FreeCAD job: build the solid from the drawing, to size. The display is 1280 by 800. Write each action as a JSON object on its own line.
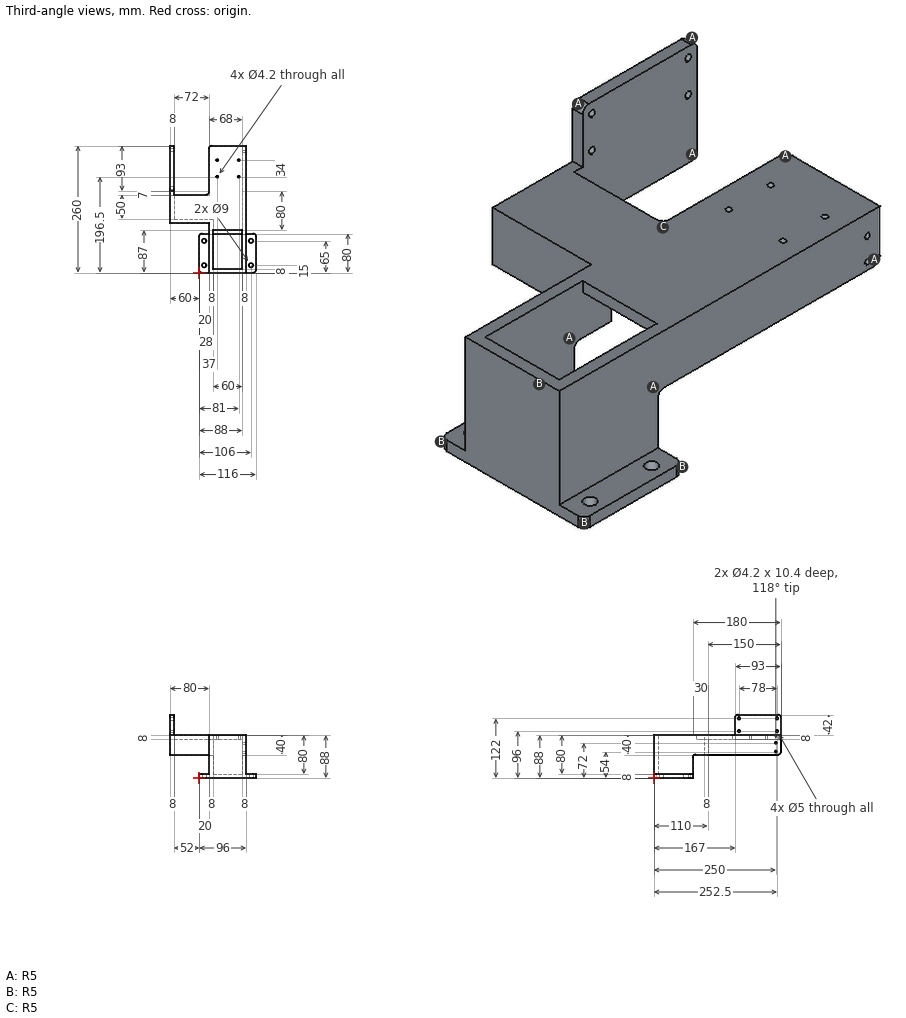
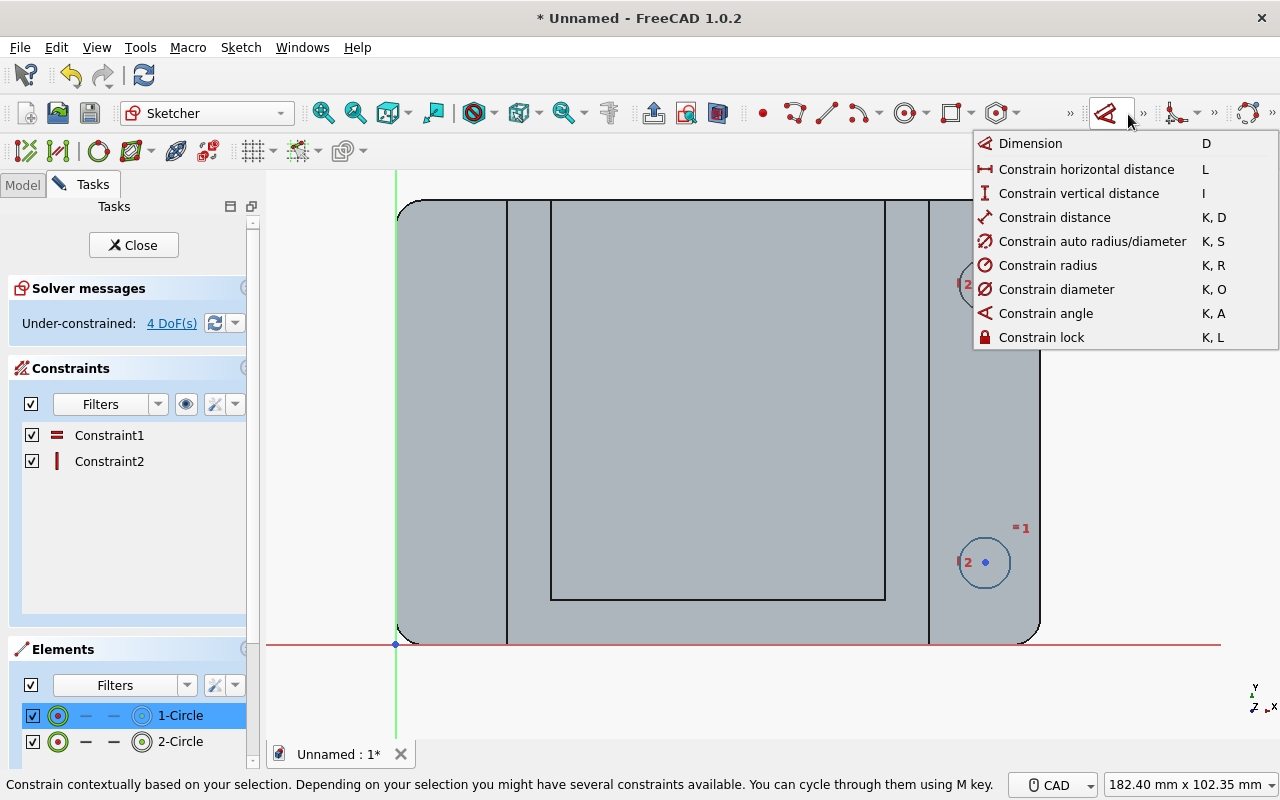
{"action": "left_click", "coordinate": [1126, 289]}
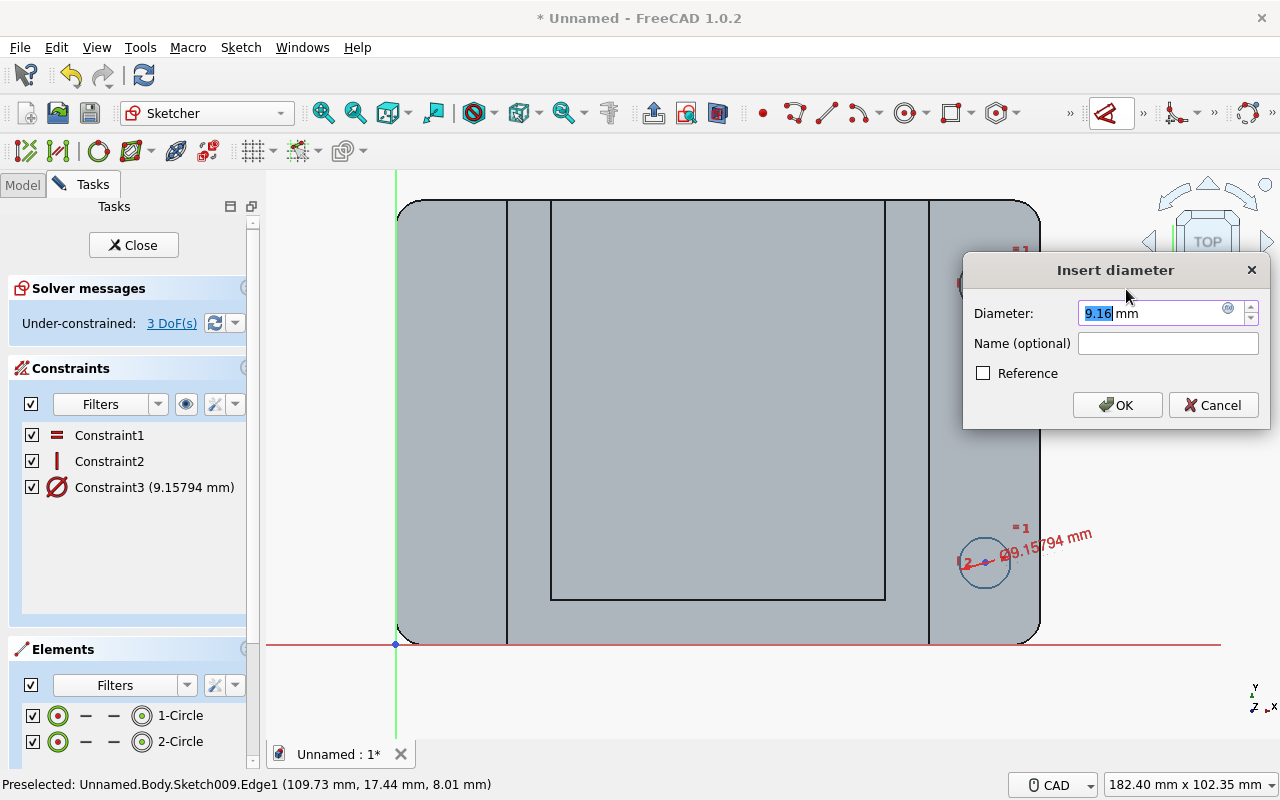
{"action": "type", "text": "9"}
{"action": "key", "text": "Return"}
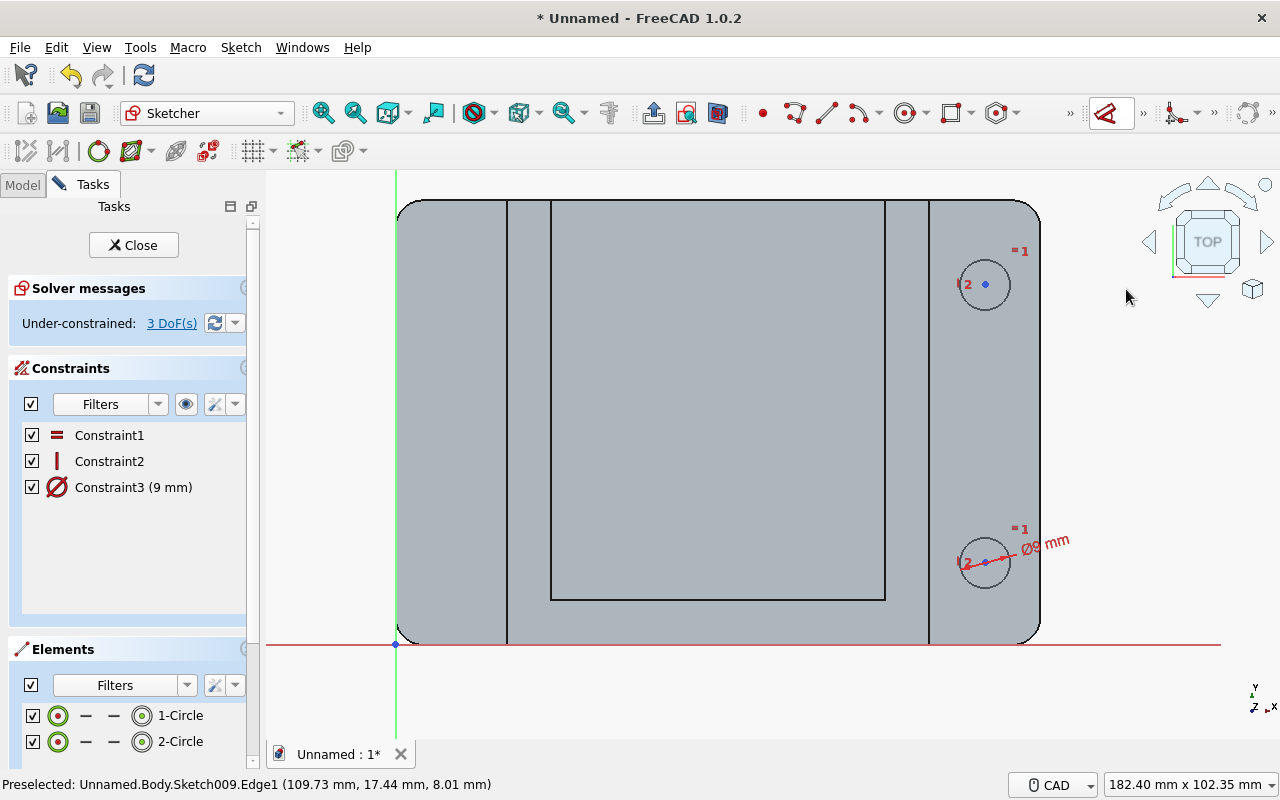
{"action": "left_click", "coordinate": [985, 563]}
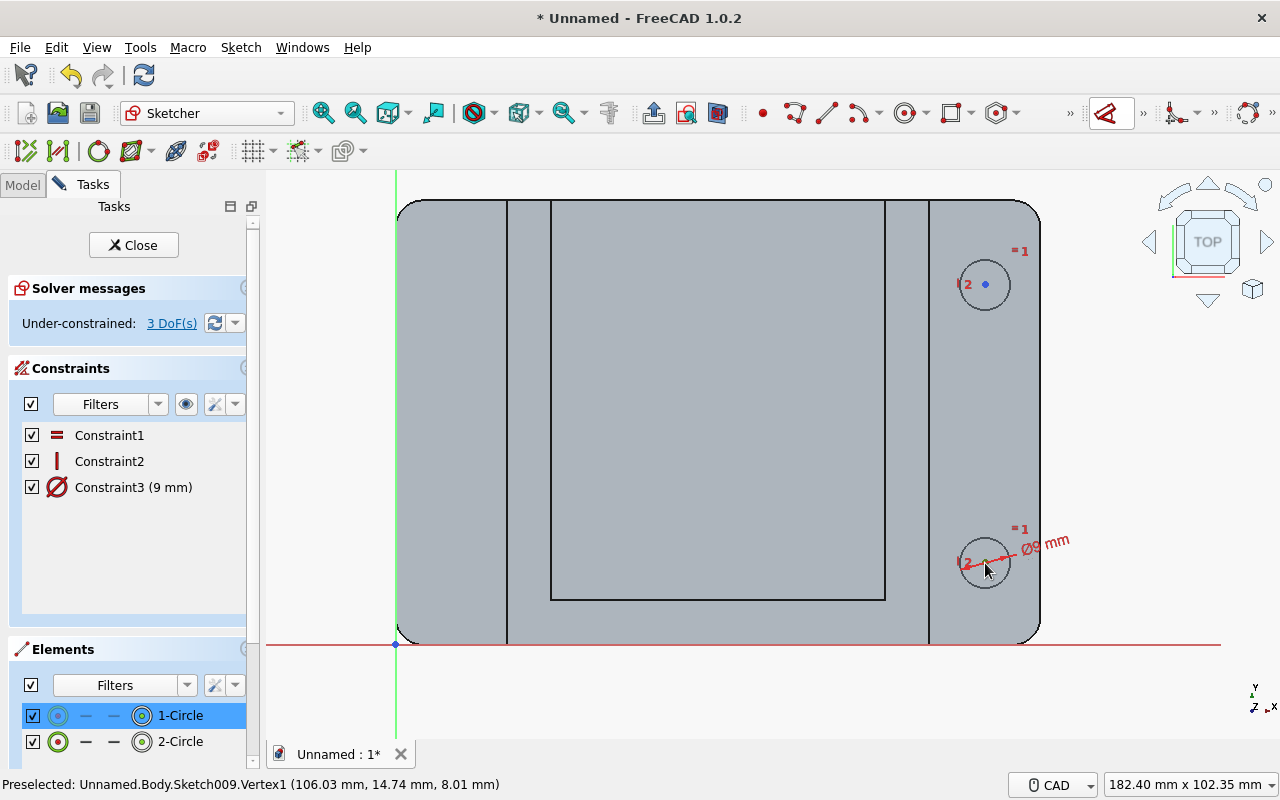
{"action": "left_click", "coordinate": [1128, 114]}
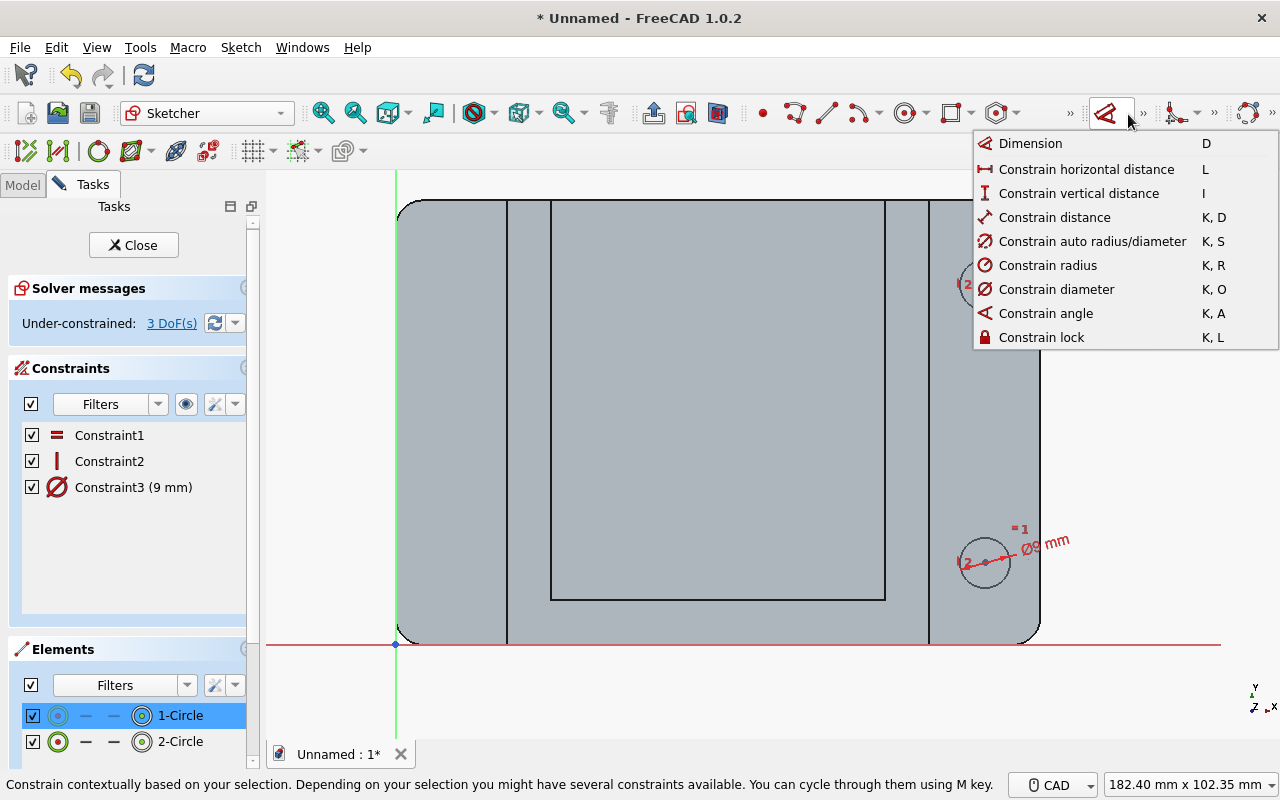
{"action": "left_click", "coordinate": [1126, 193]}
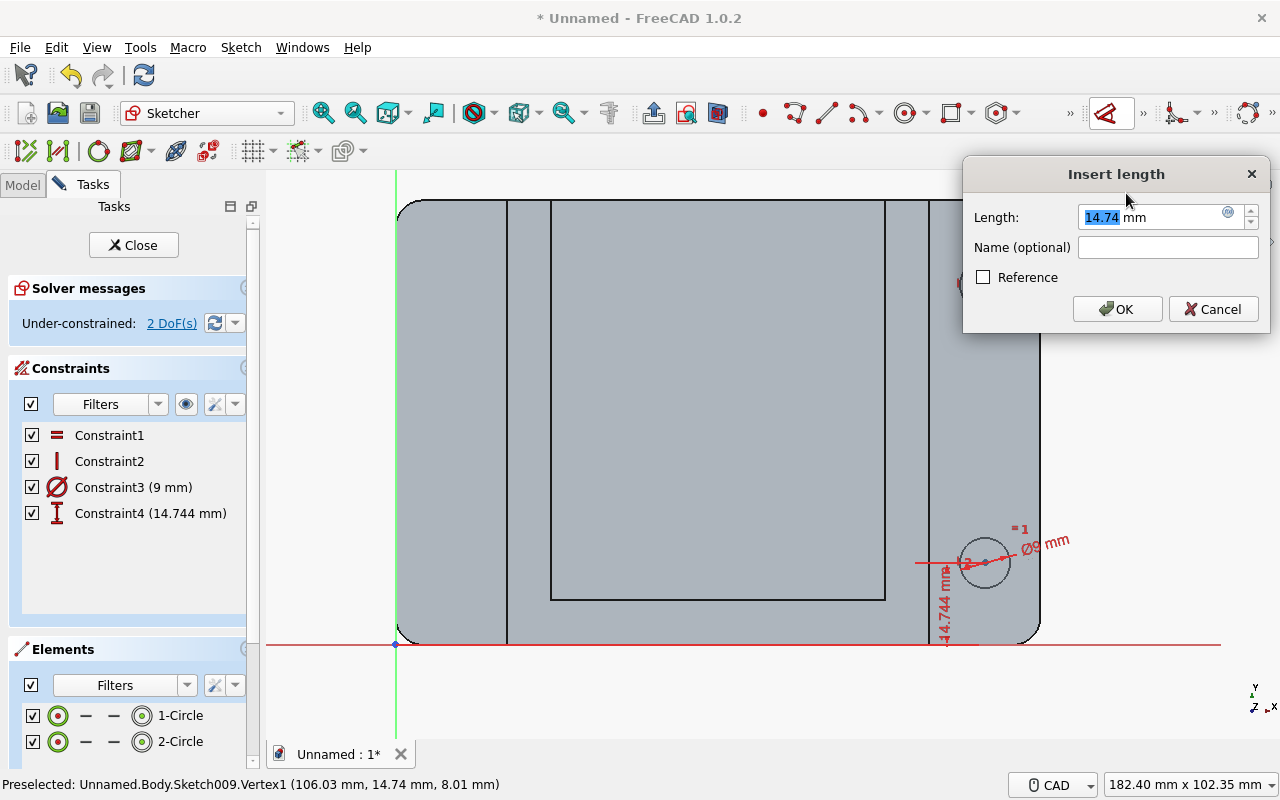
{"action": "type", "text": "15"}
{"action": "key", "text": "Return"}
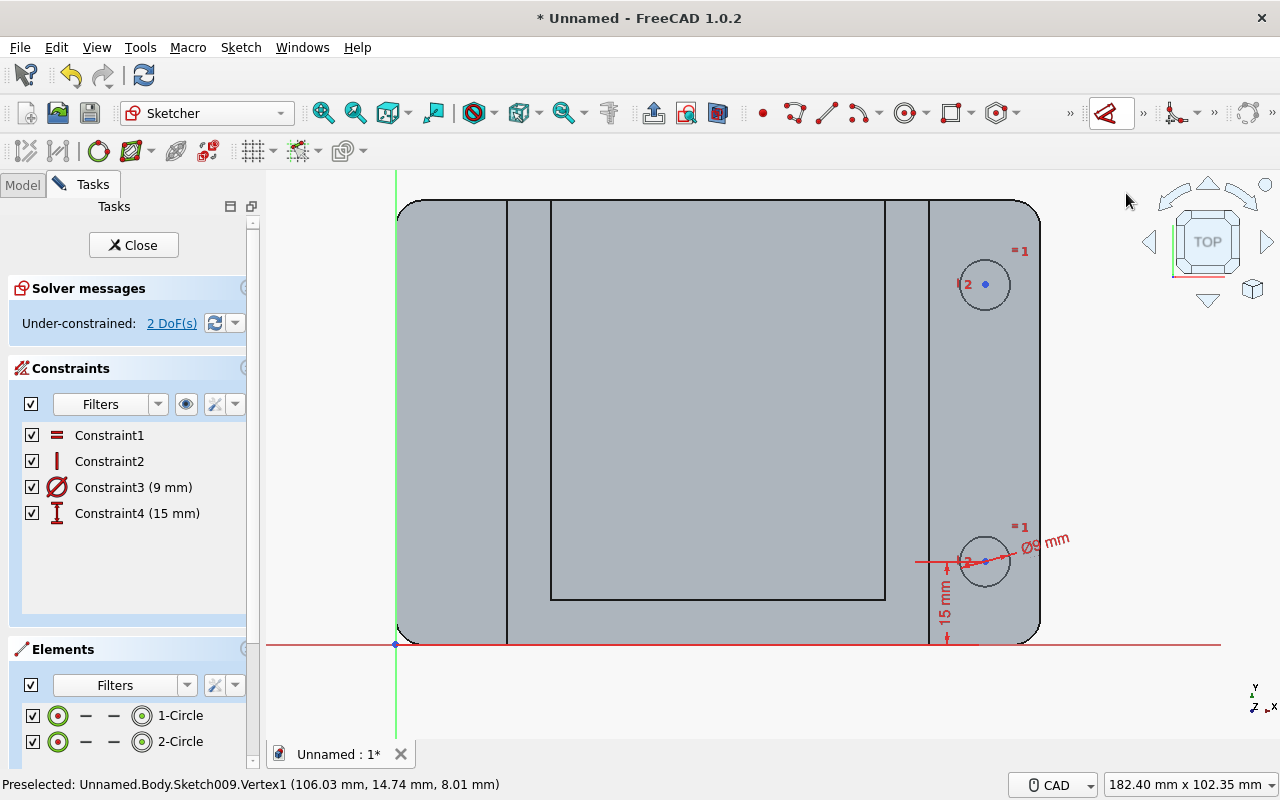
{"action": "left_click", "coordinate": [985, 285]}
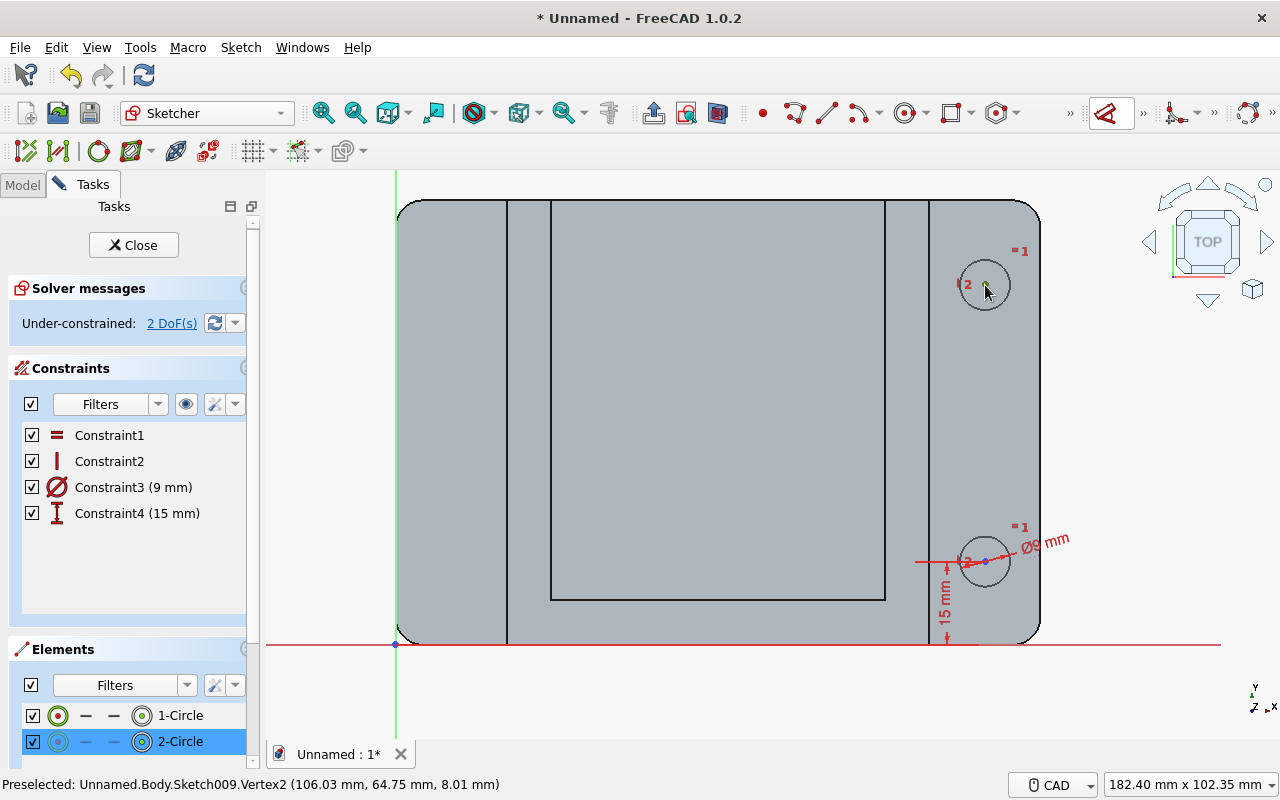
{"action": "key", "text": "i"}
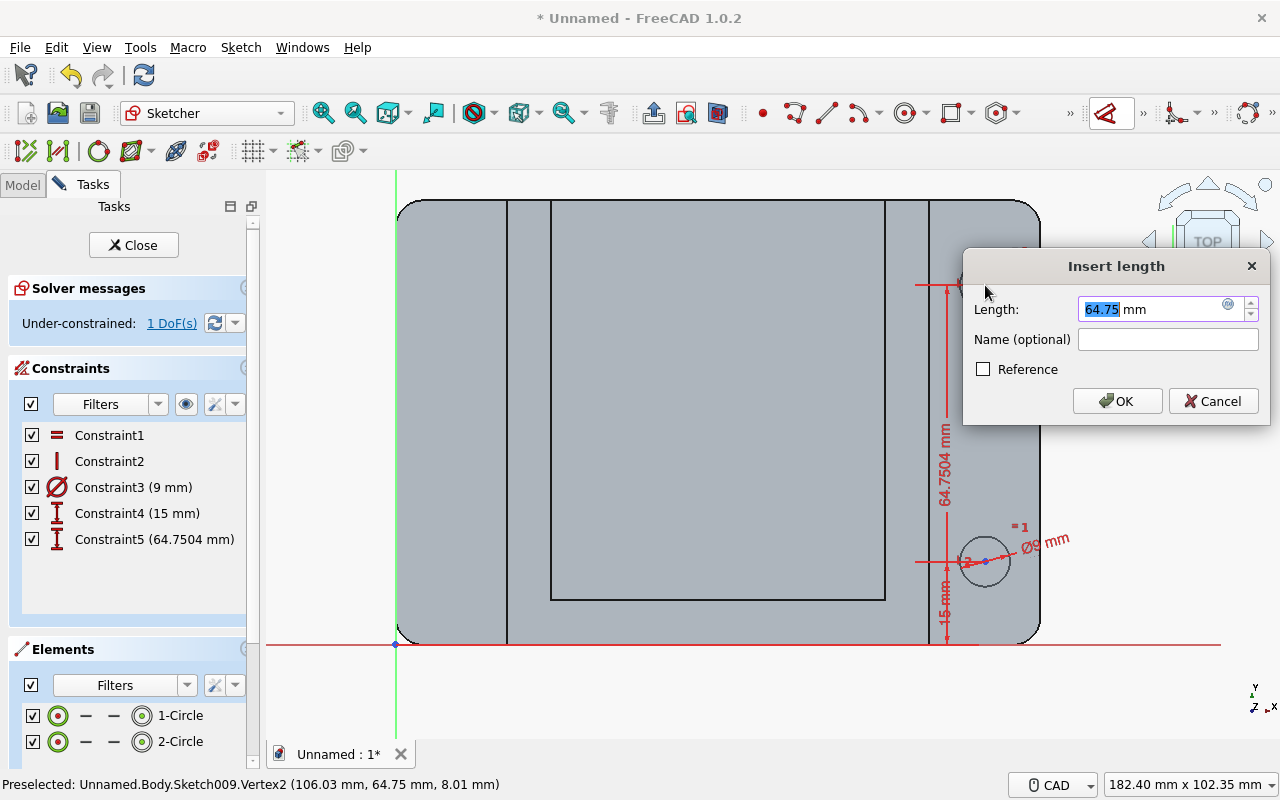
{"action": "type", "text": "65"}
{"action": "key", "text": "Return"}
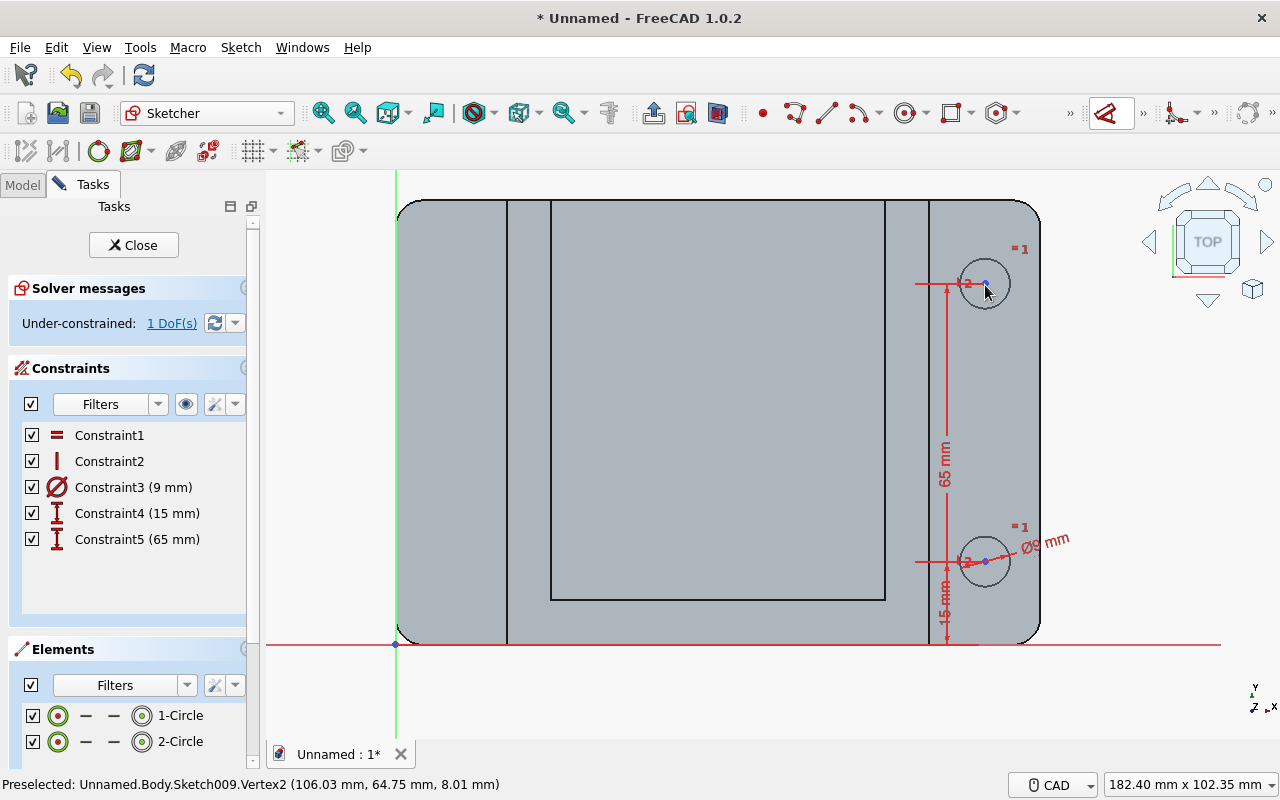
{"action": "left_click", "coordinate": [985, 562]}